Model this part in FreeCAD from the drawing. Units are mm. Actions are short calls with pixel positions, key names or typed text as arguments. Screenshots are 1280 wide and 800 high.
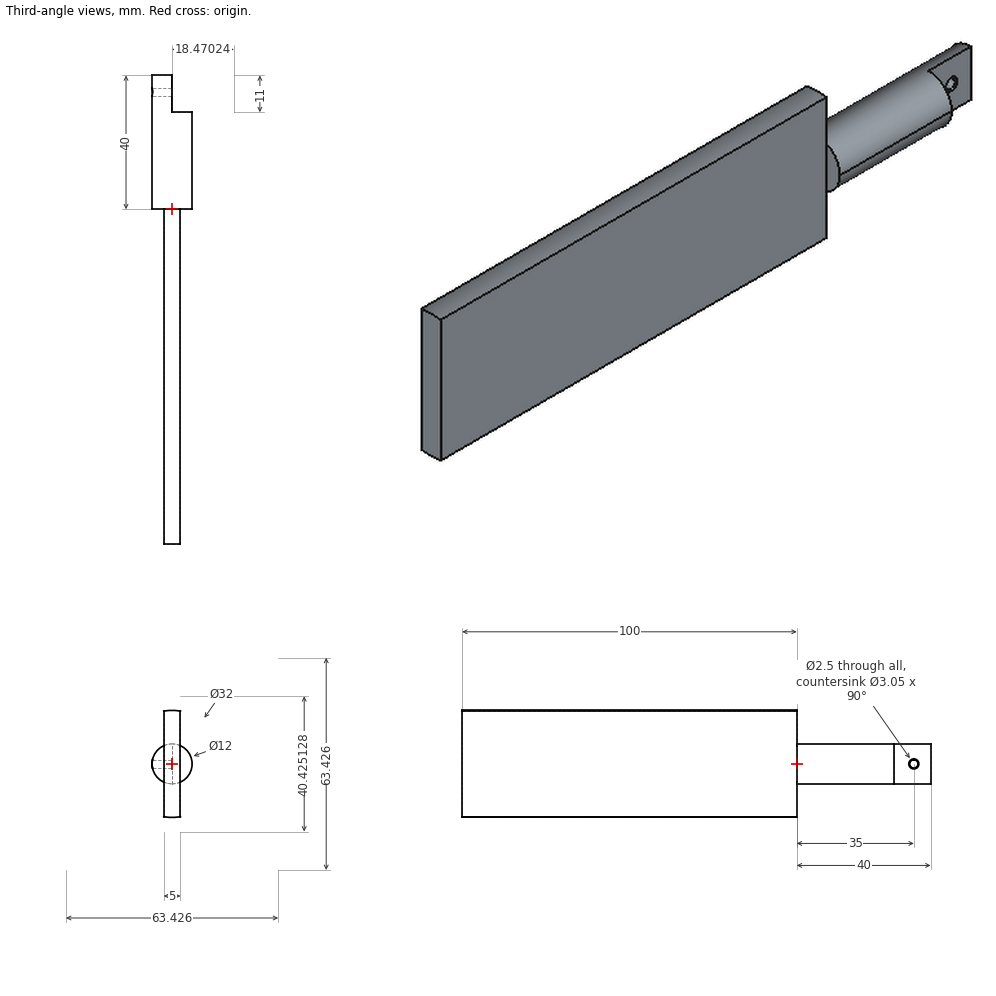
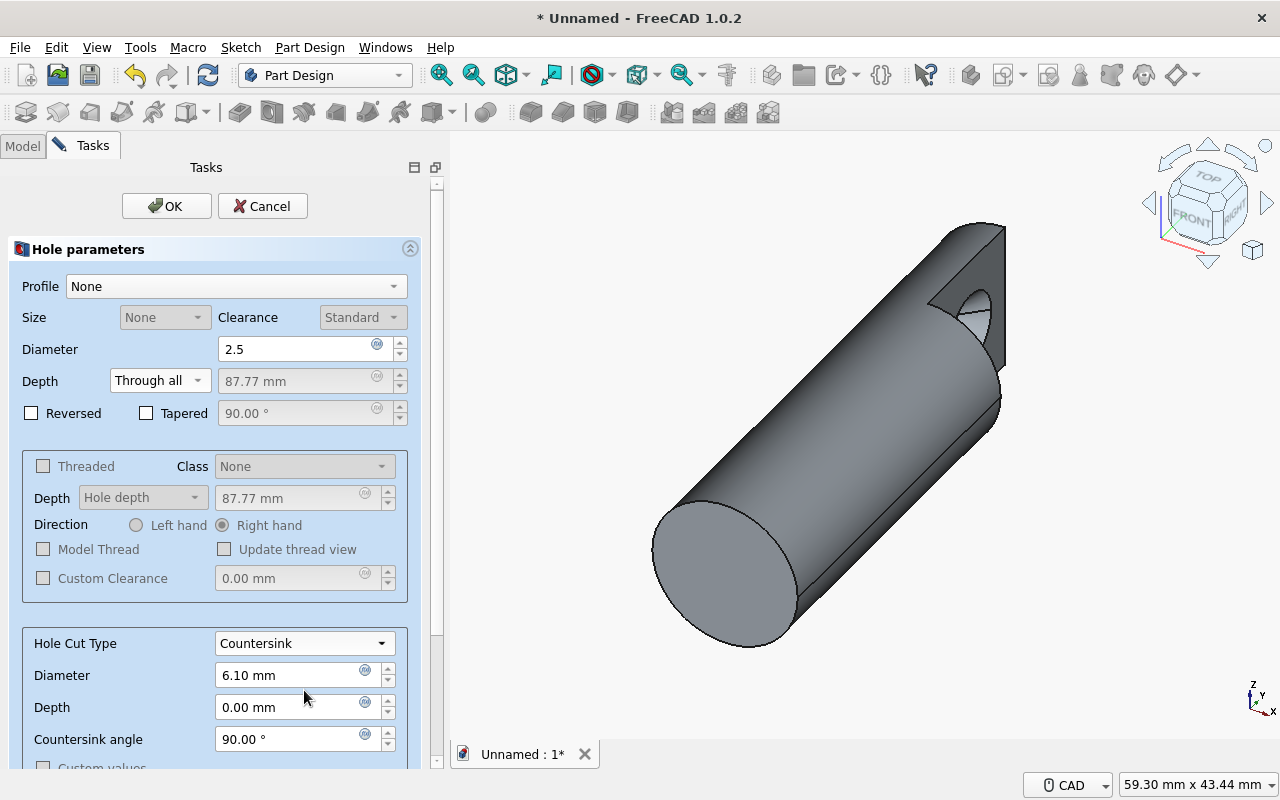
triple_click(298, 675)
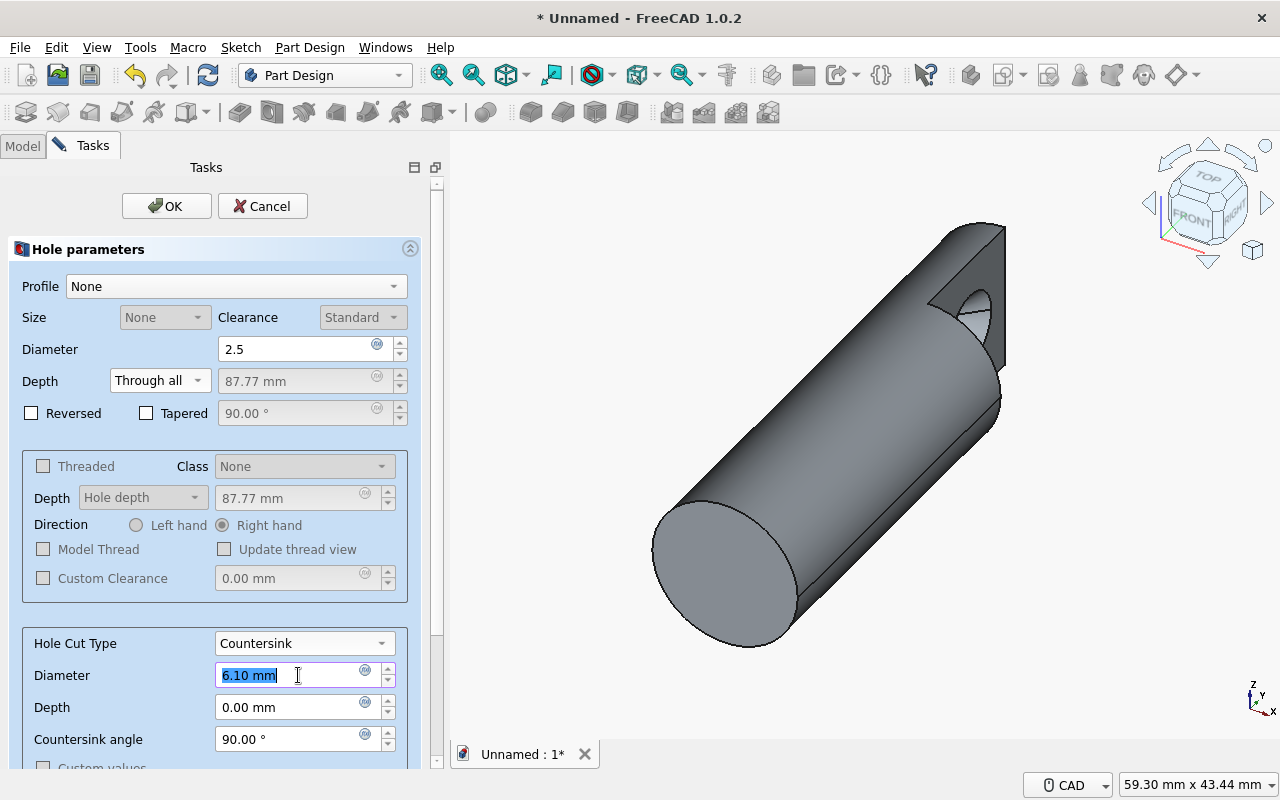
text(3.05)
key(Tab)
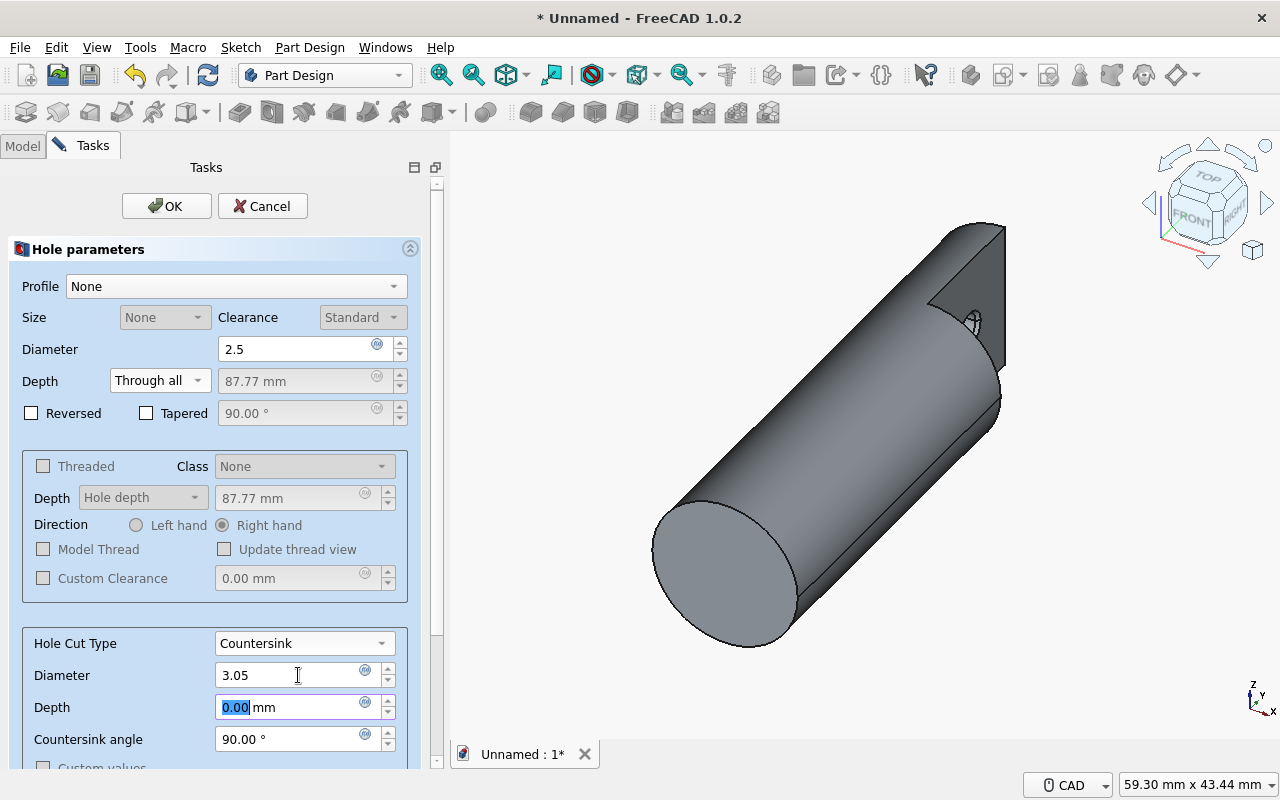
click(167, 206)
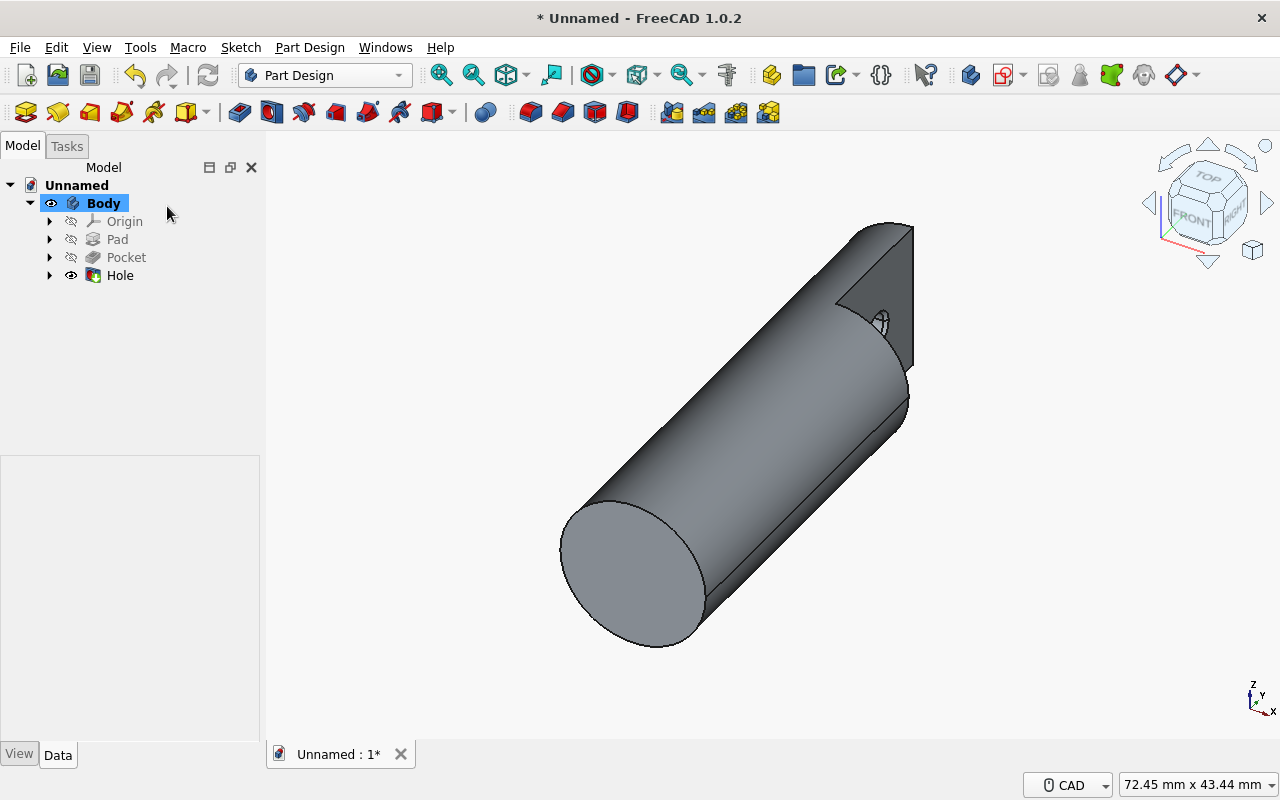
click(633, 573)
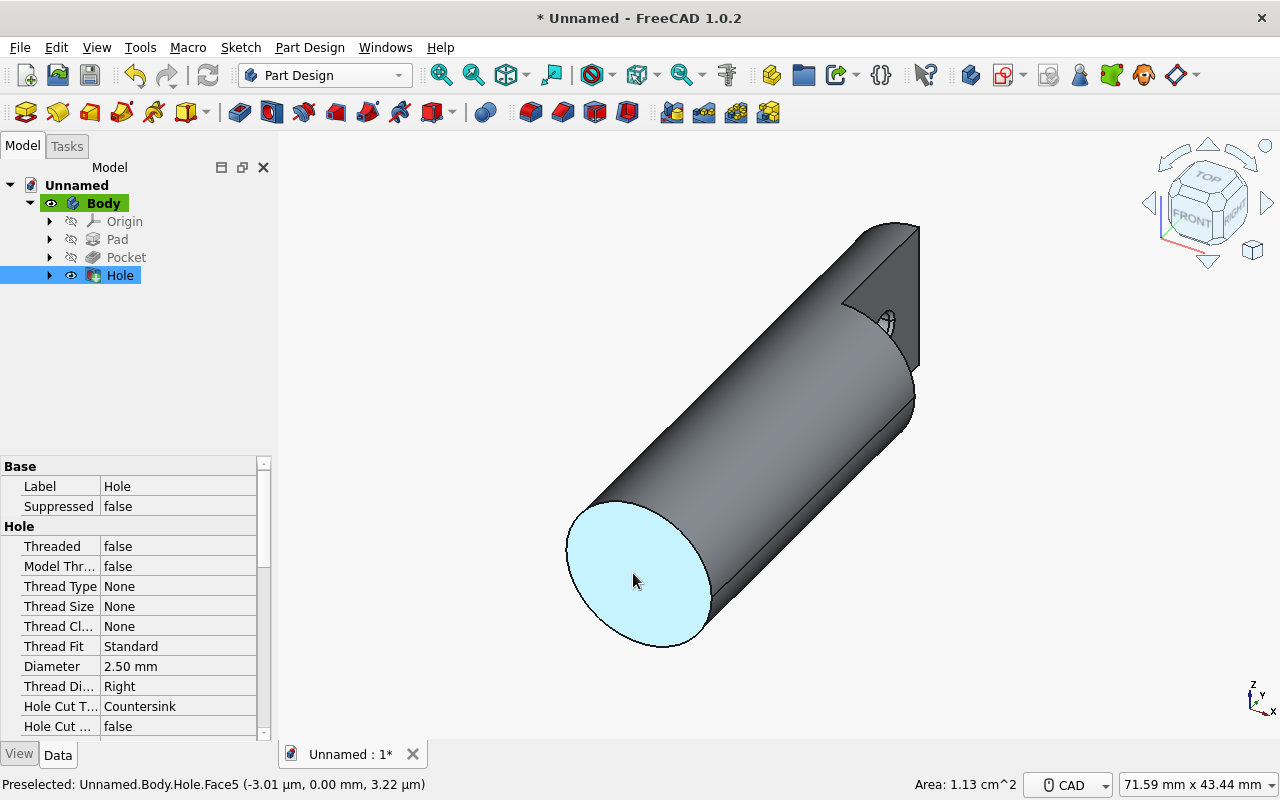
click(1004, 76)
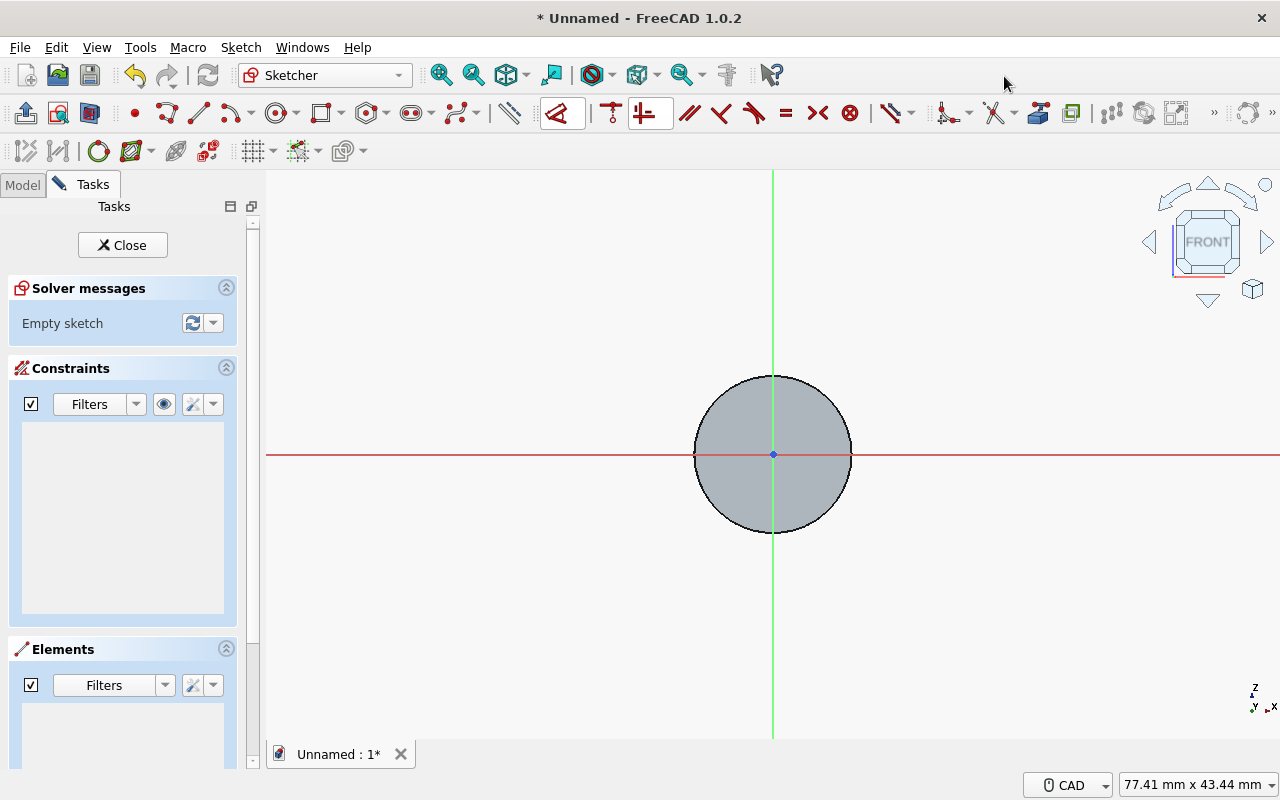
click(276, 114)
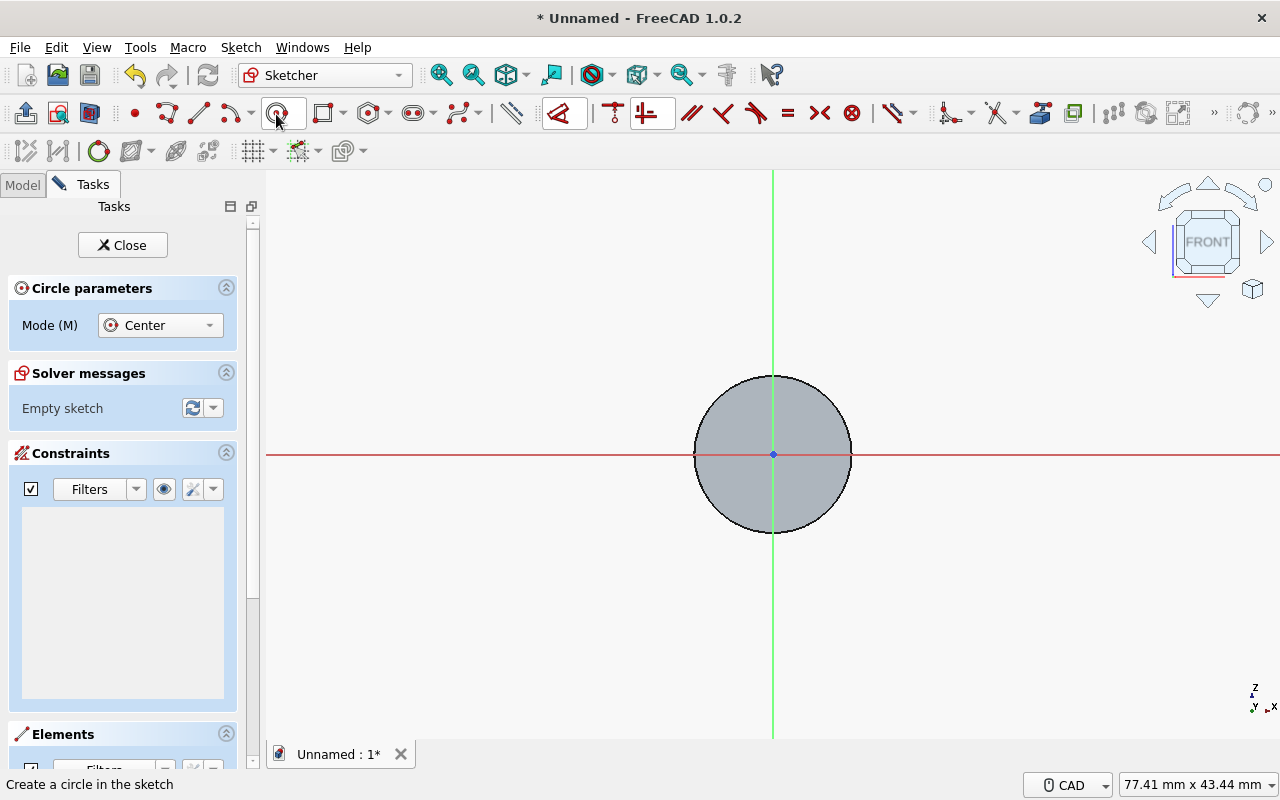
click(773, 455)
move(921, 306)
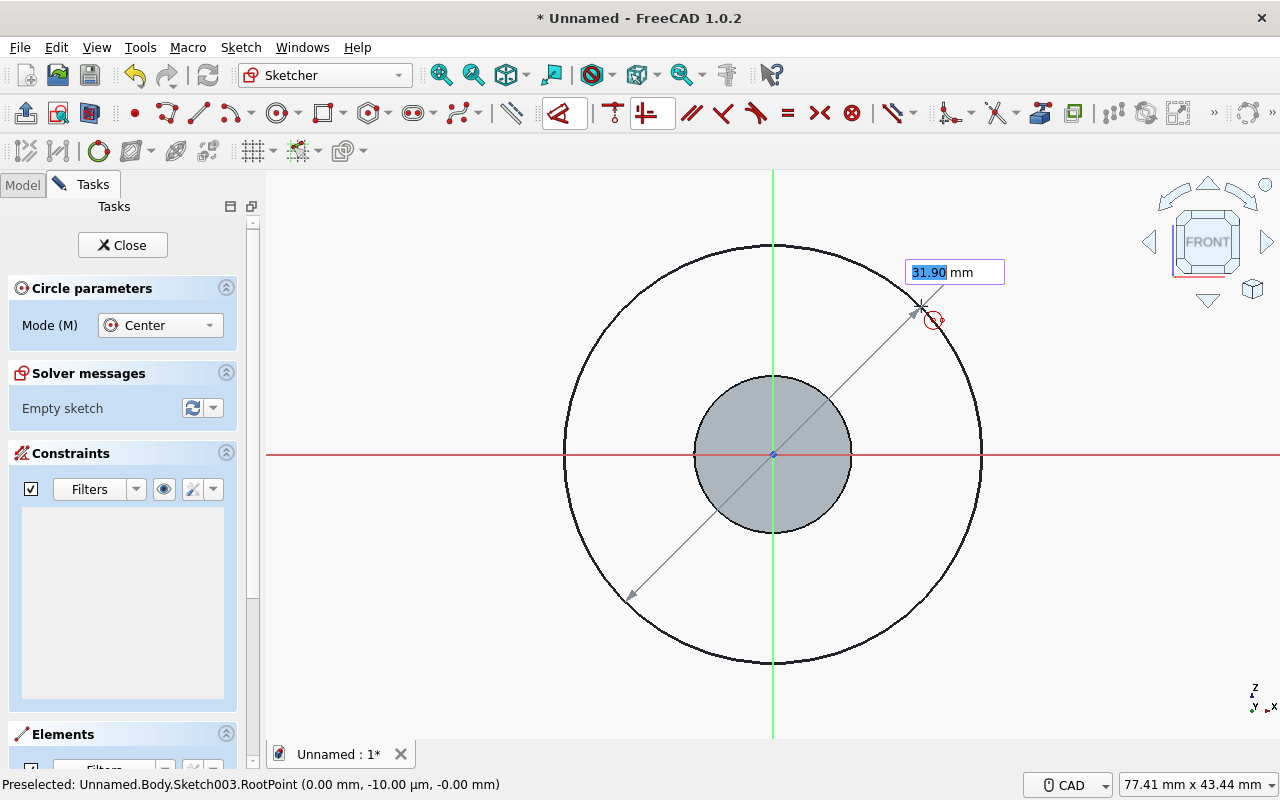
text(32)
key(Return)
key(Escape)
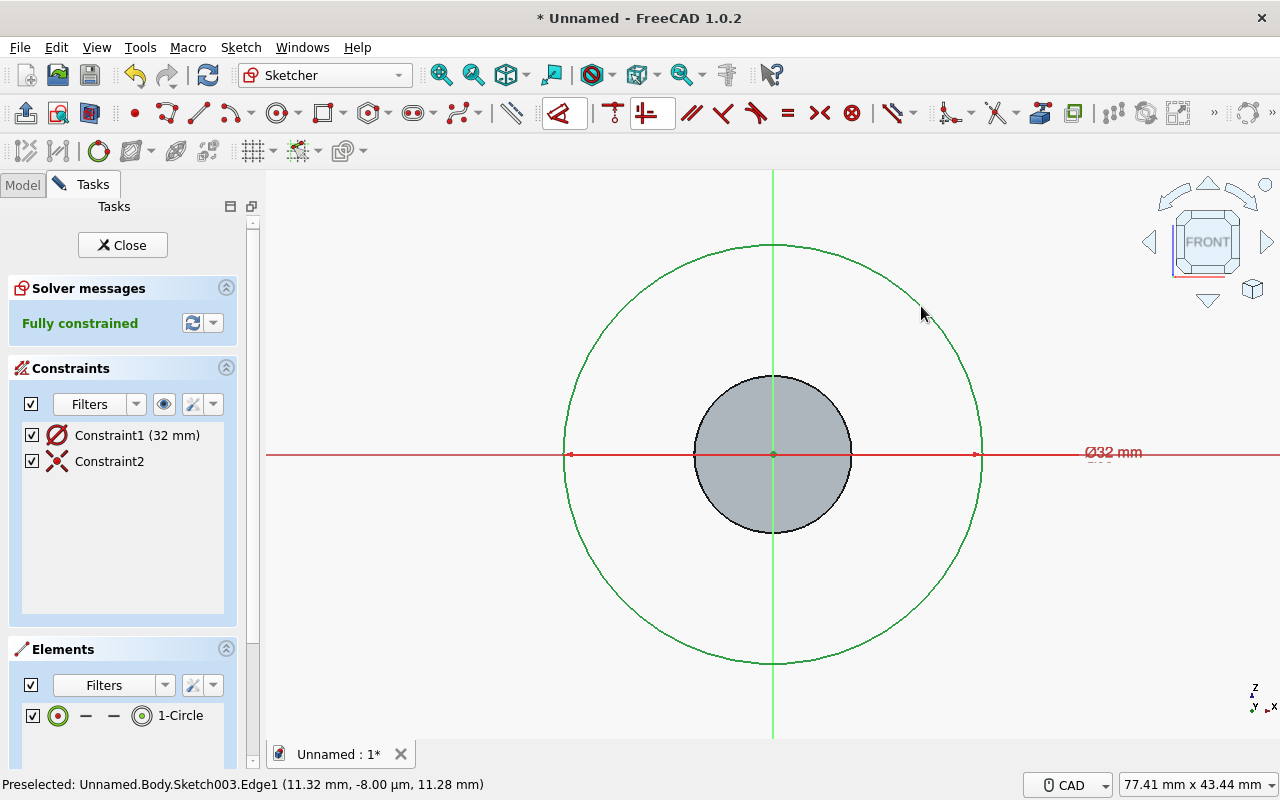
click(123, 245)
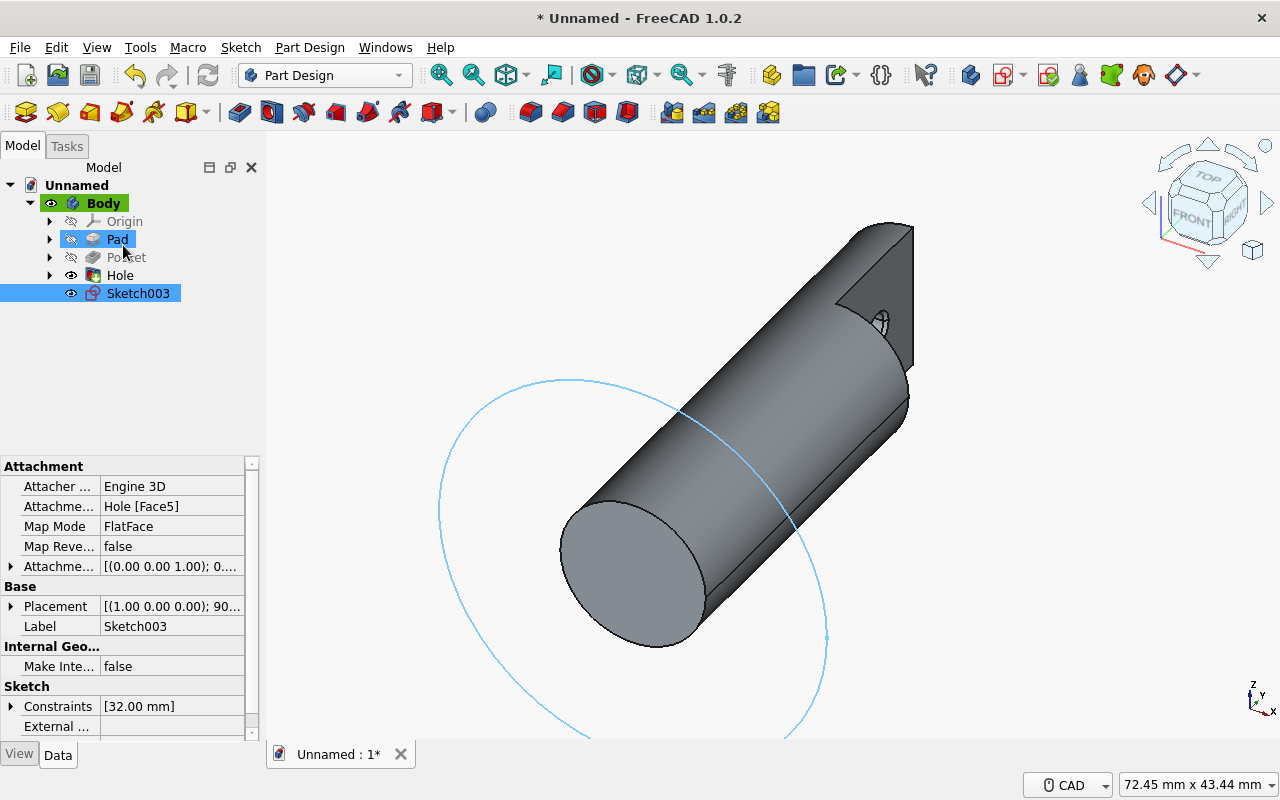
click(26, 112)